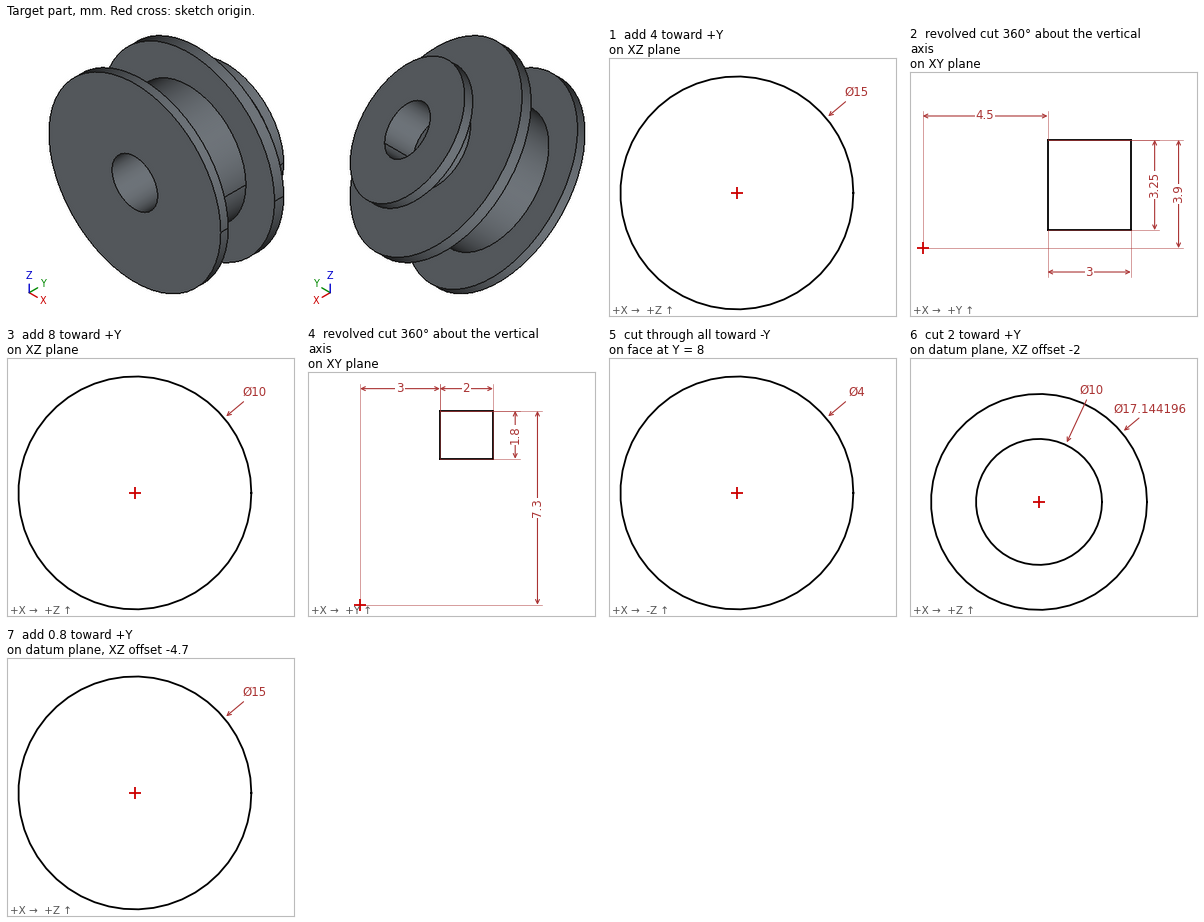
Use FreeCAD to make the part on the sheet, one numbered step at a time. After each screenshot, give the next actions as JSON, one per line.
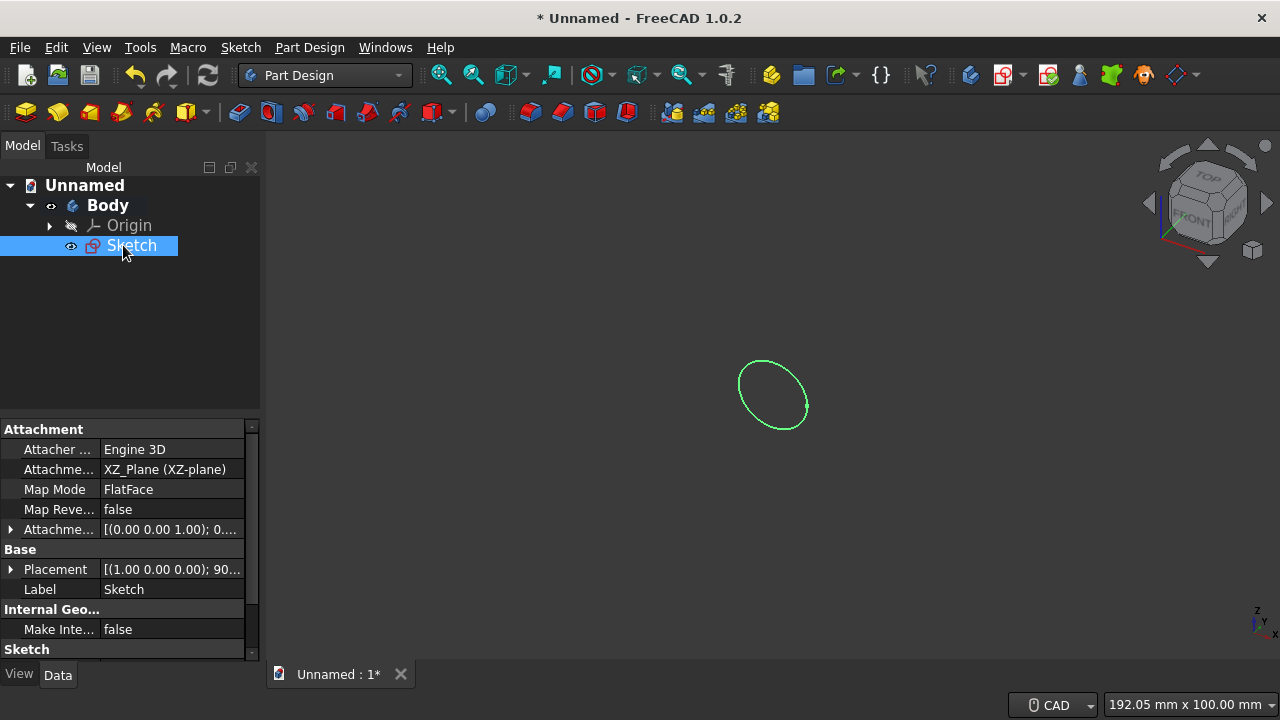
{"action": "left_click", "coordinate": [26, 112]}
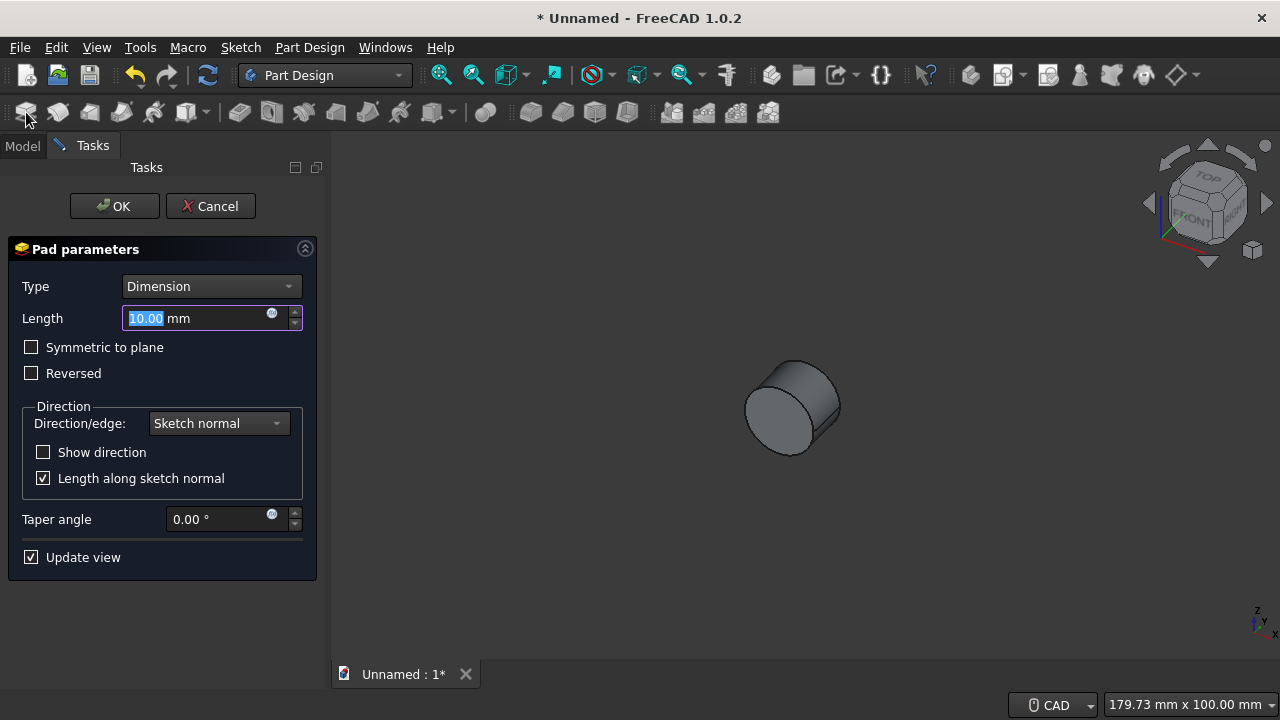
{"action": "type", "text": "4"}
{"action": "key", "text": "Tab"}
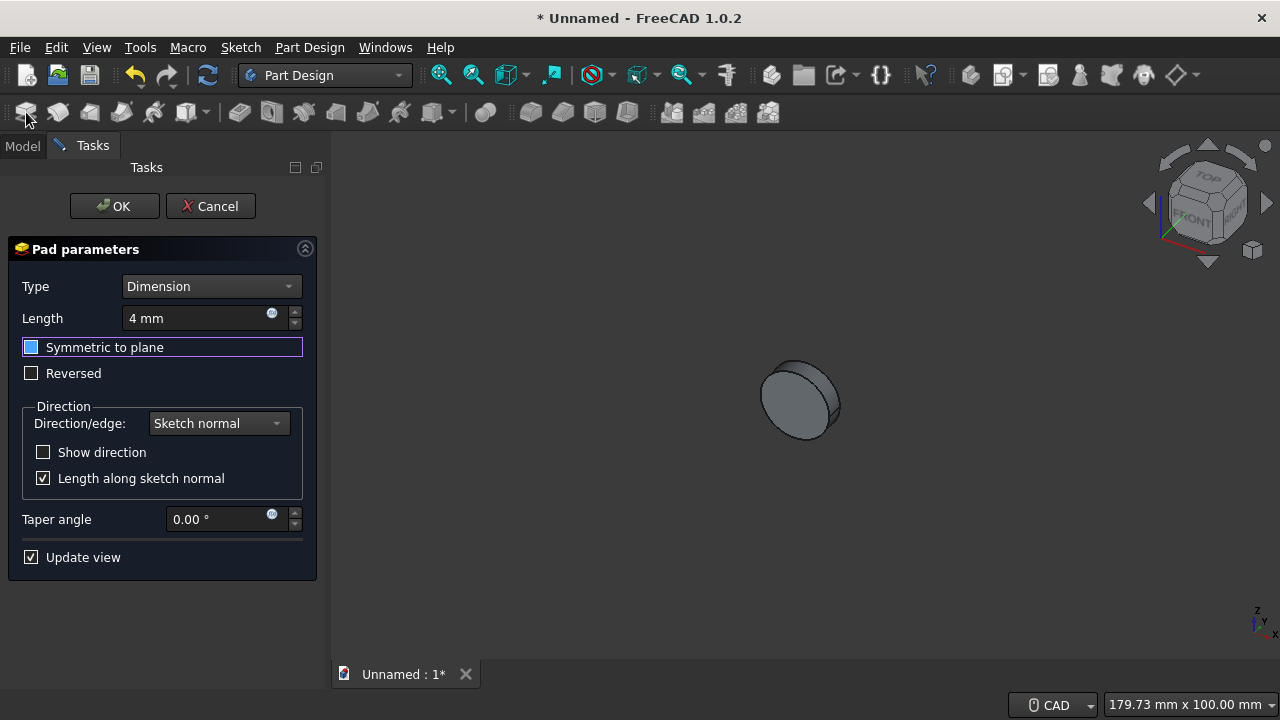
{"action": "left_click", "coordinate": [30, 373]}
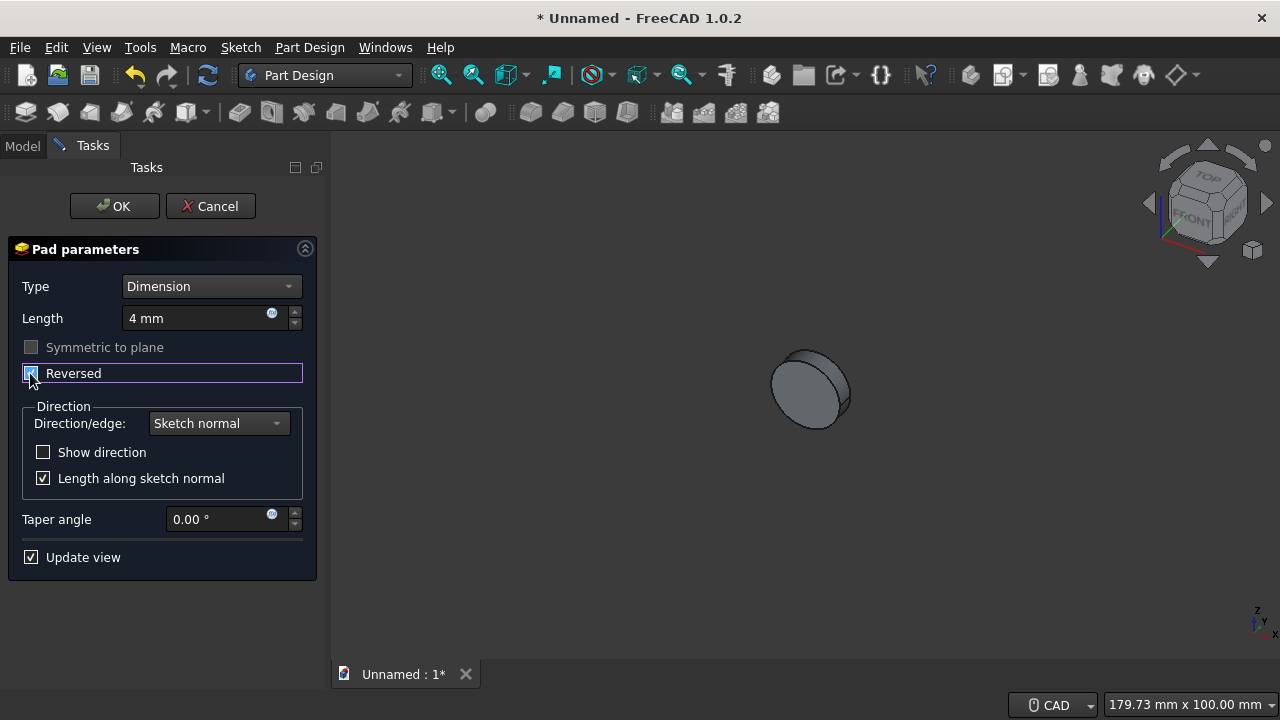
{"action": "left_click", "coordinate": [115, 206]}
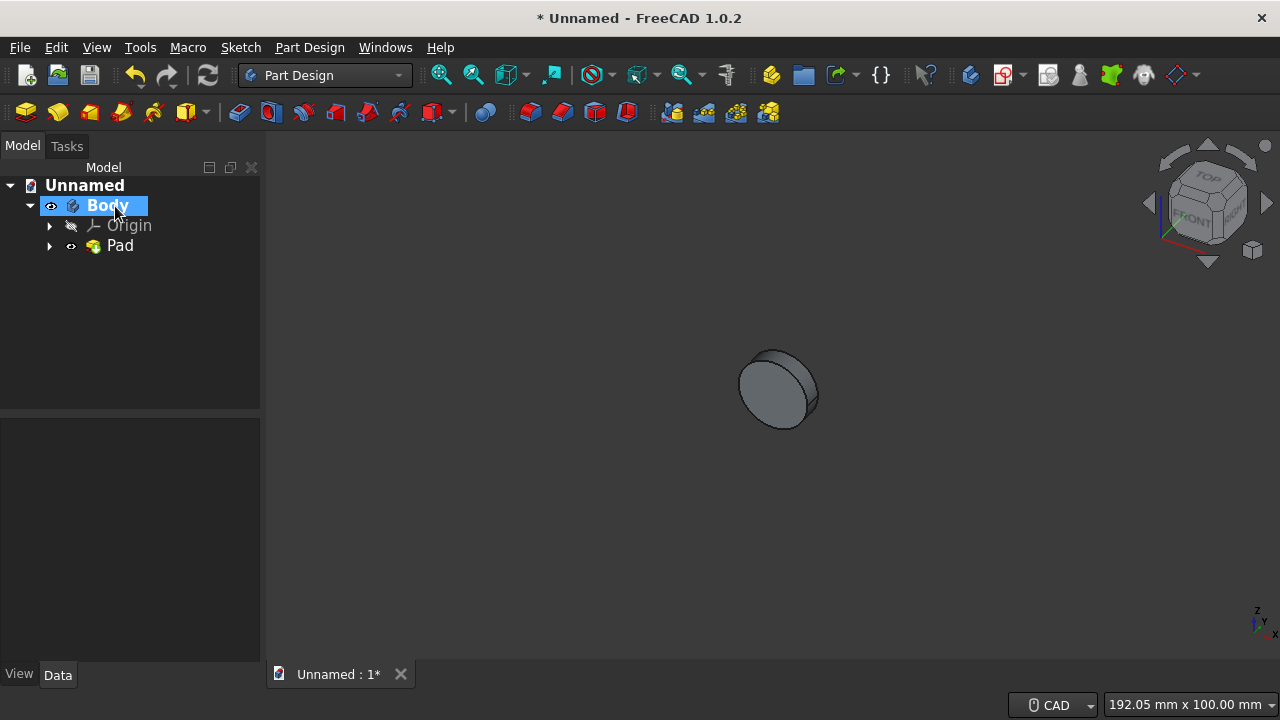
{"action": "left_click", "coordinate": [442, 76]}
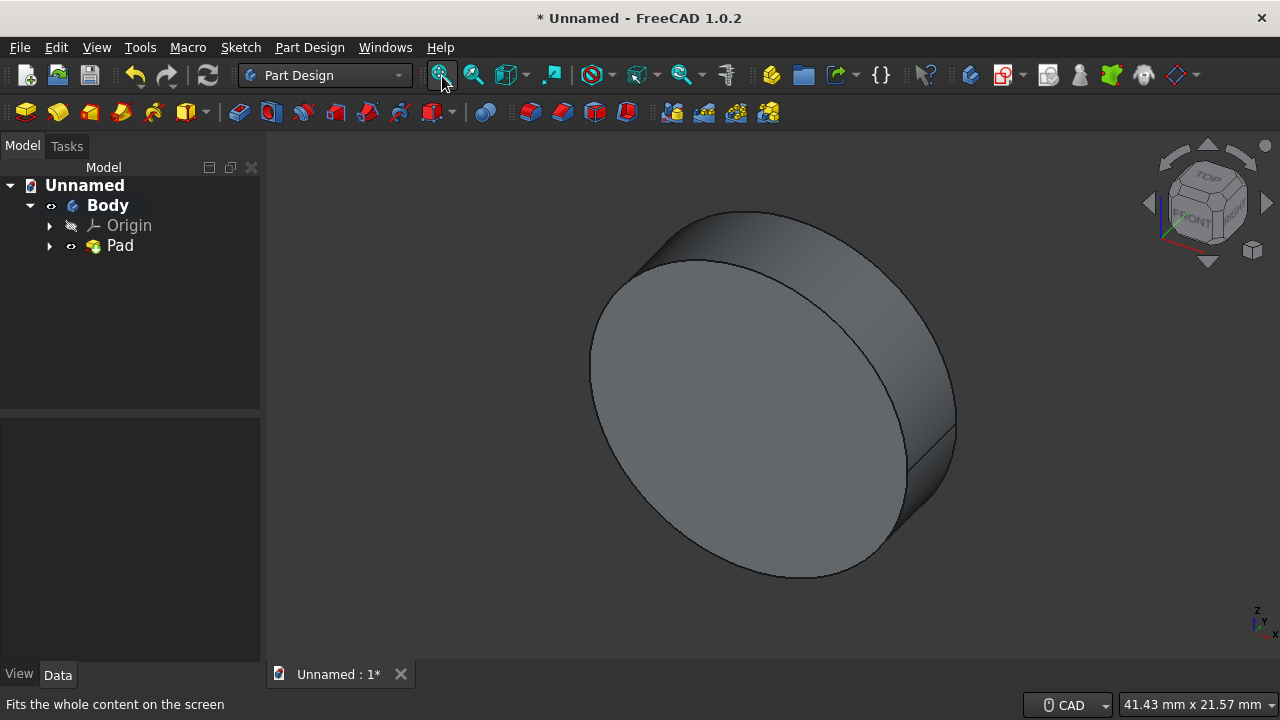
{"action": "left_click", "coordinate": [1004, 76]}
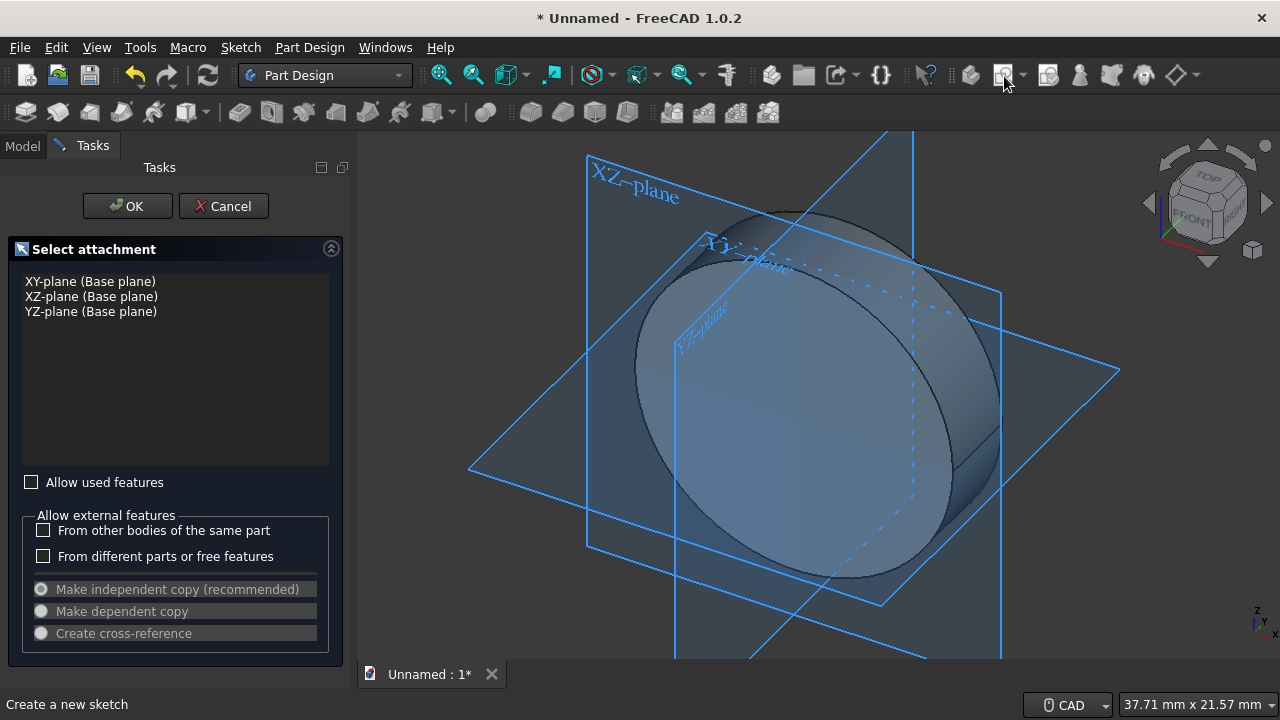
{"action": "left_click", "coordinate": [82, 282]}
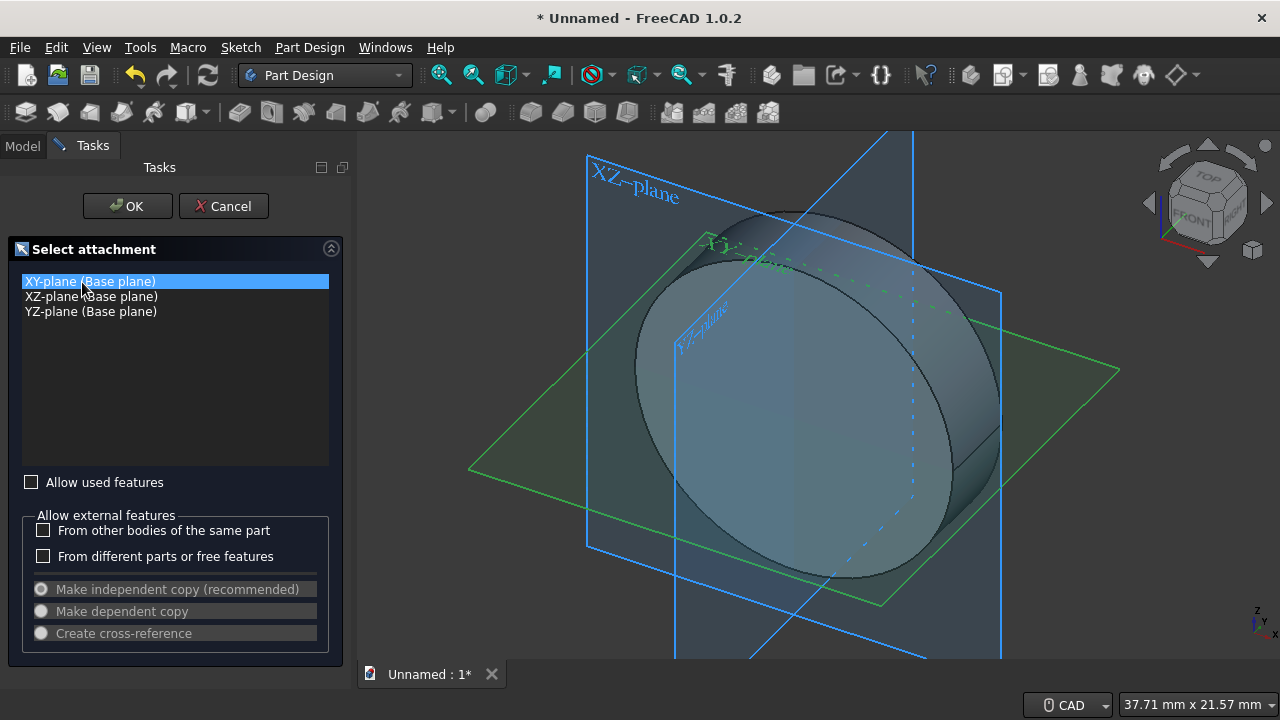
{"action": "left_click", "coordinate": [128, 206]}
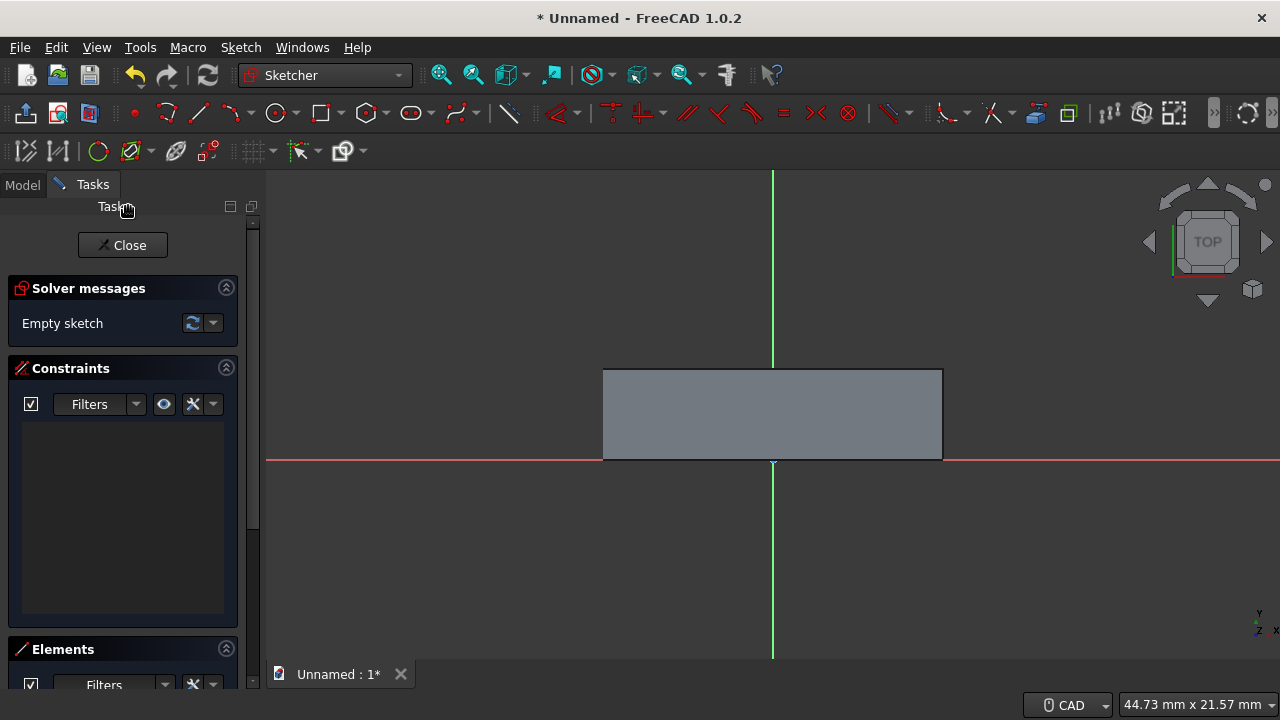
{"action": "key", "text": "q s"}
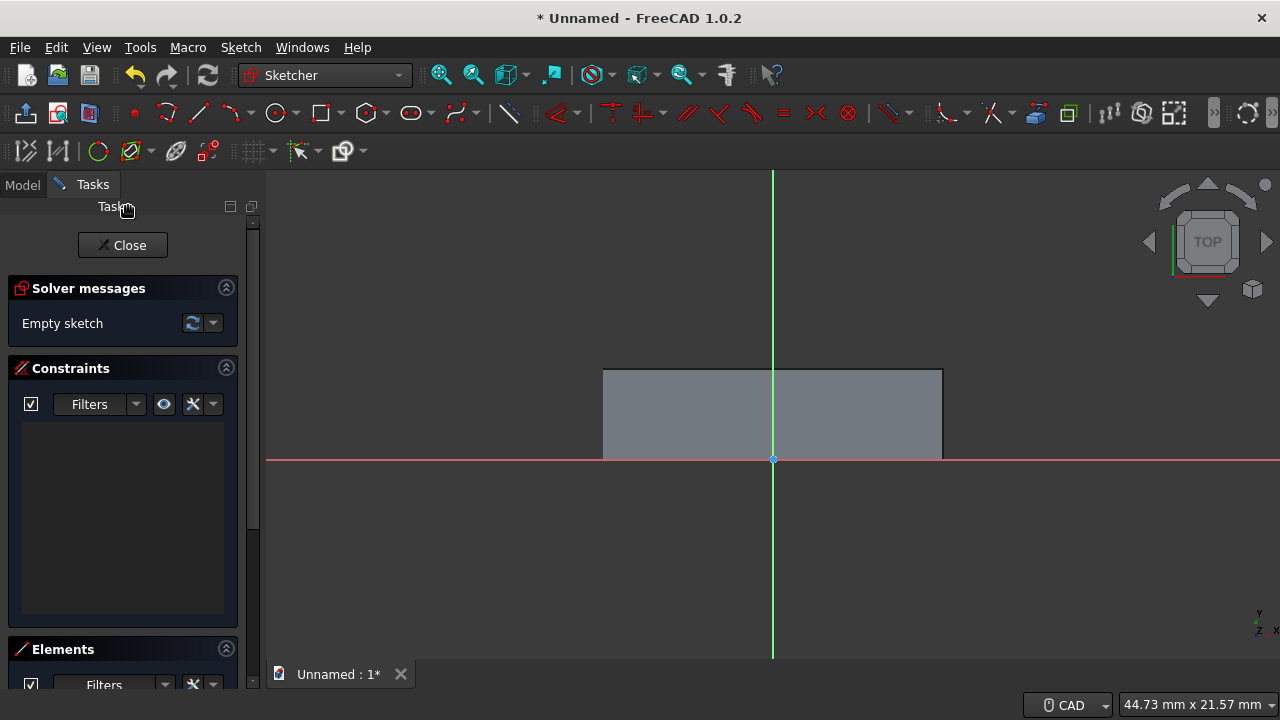
{"action": "scroll", "coordinate": [924, 416], "scroll_direction": "up", "scroll_amount": 6}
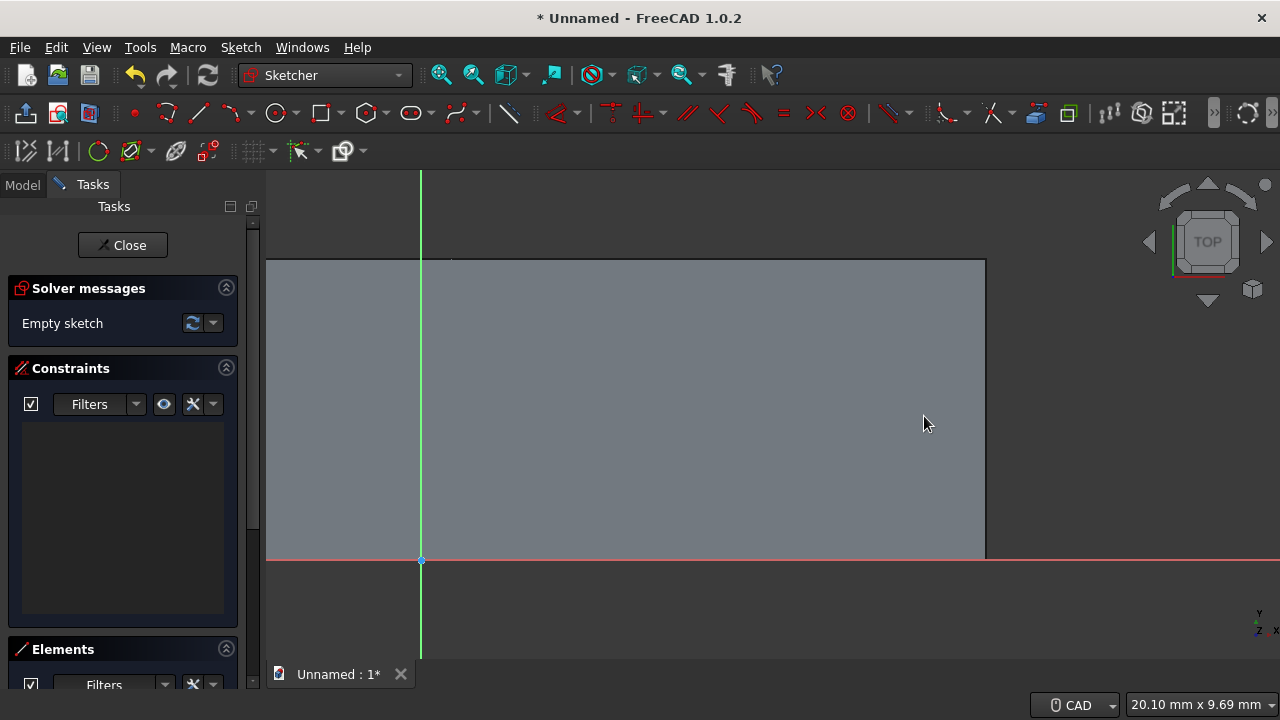
{"action": "key", "text": "g r"}